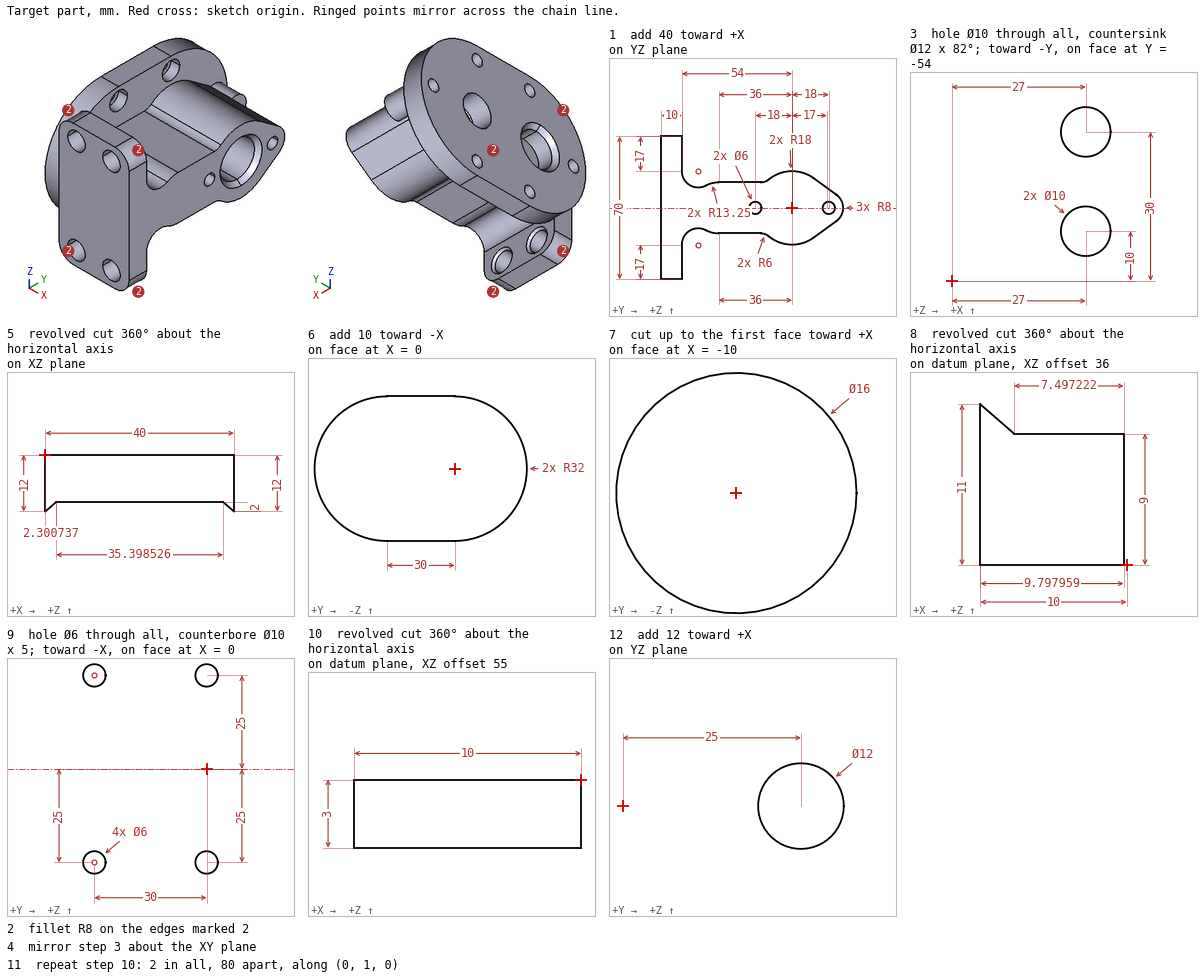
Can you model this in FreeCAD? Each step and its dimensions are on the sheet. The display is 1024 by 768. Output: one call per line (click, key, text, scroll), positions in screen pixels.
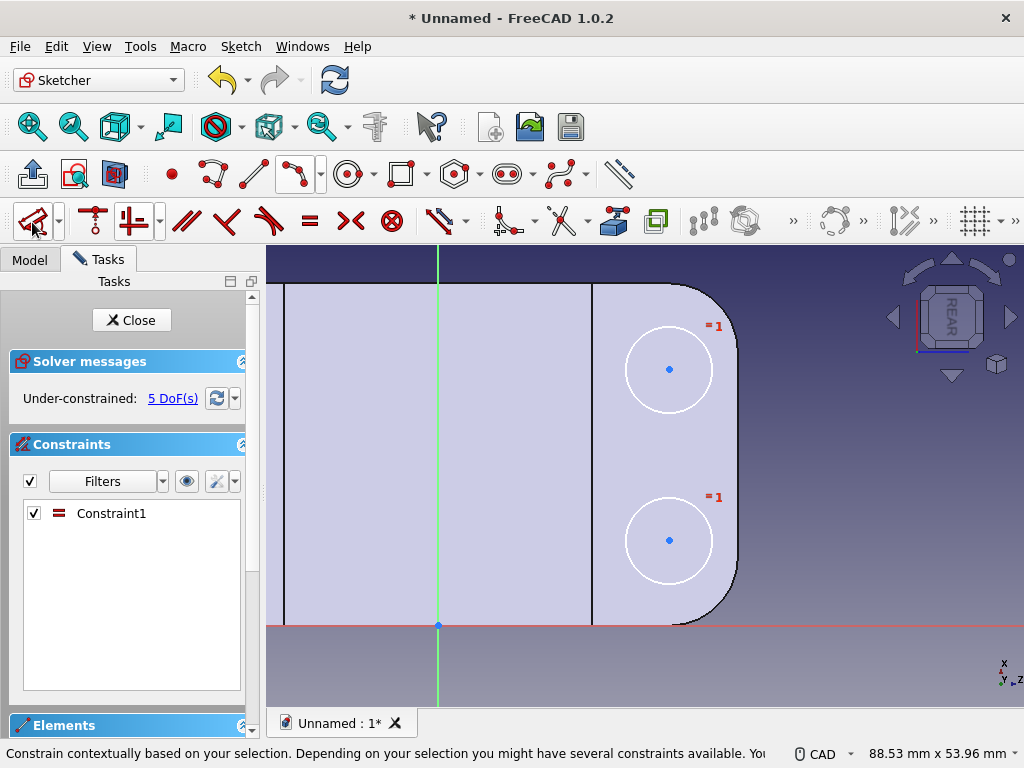
click(699, 510)
click(721, 487)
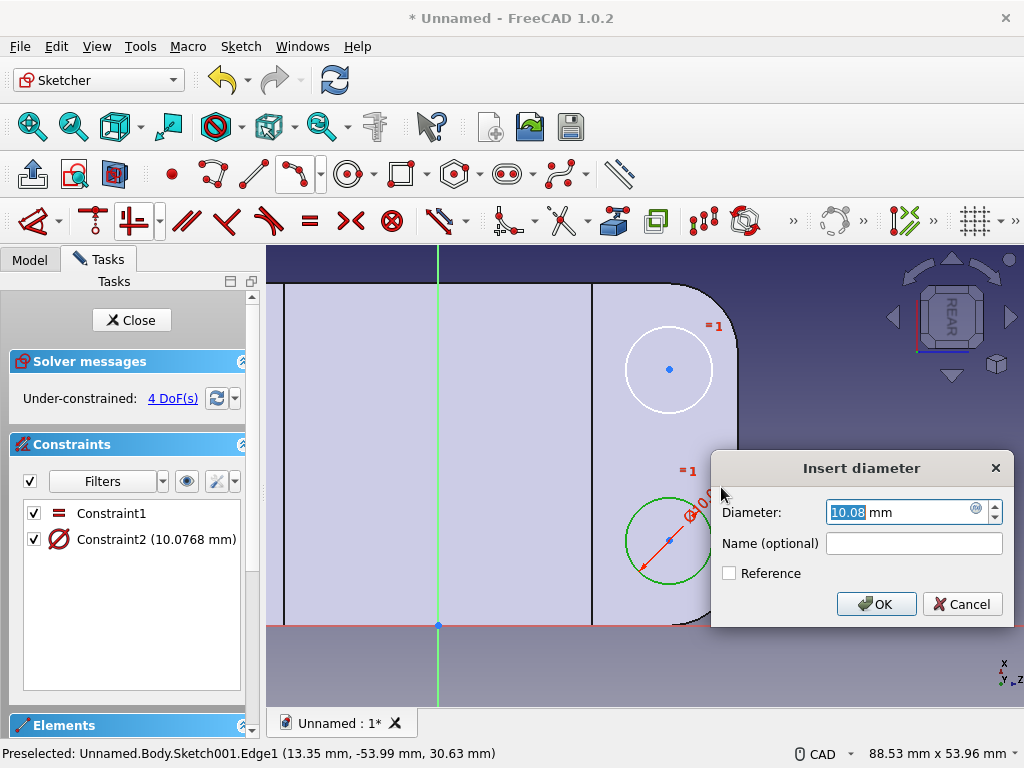
text(10)
key(Return)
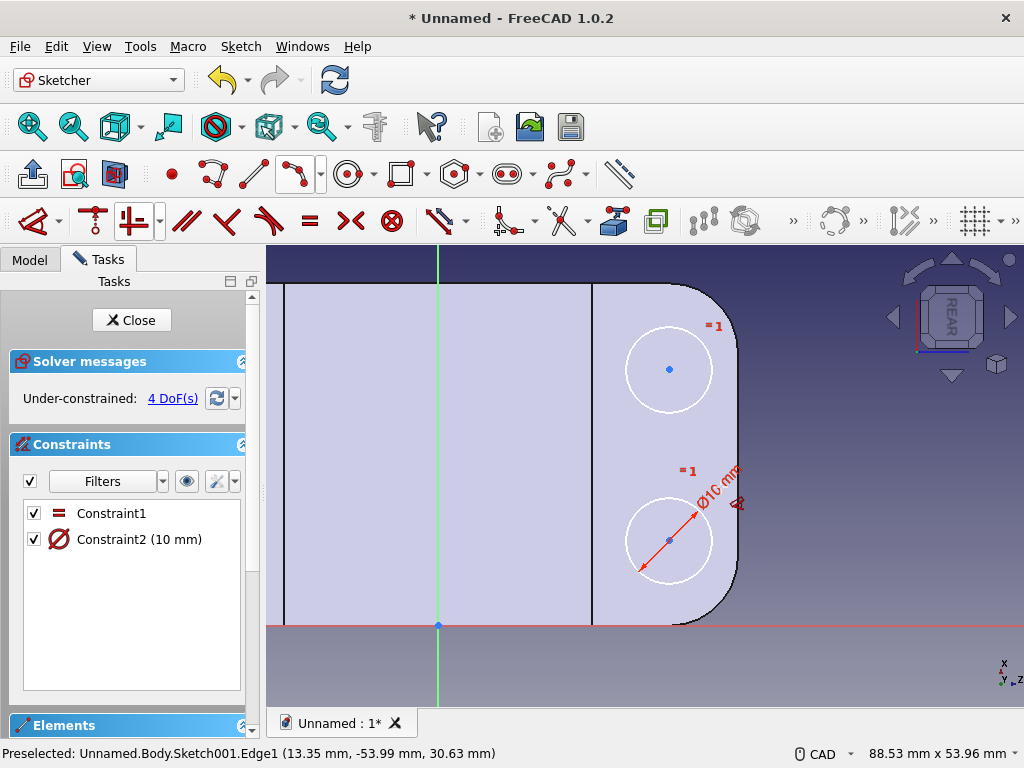
click(669, 541)
click(554, 660)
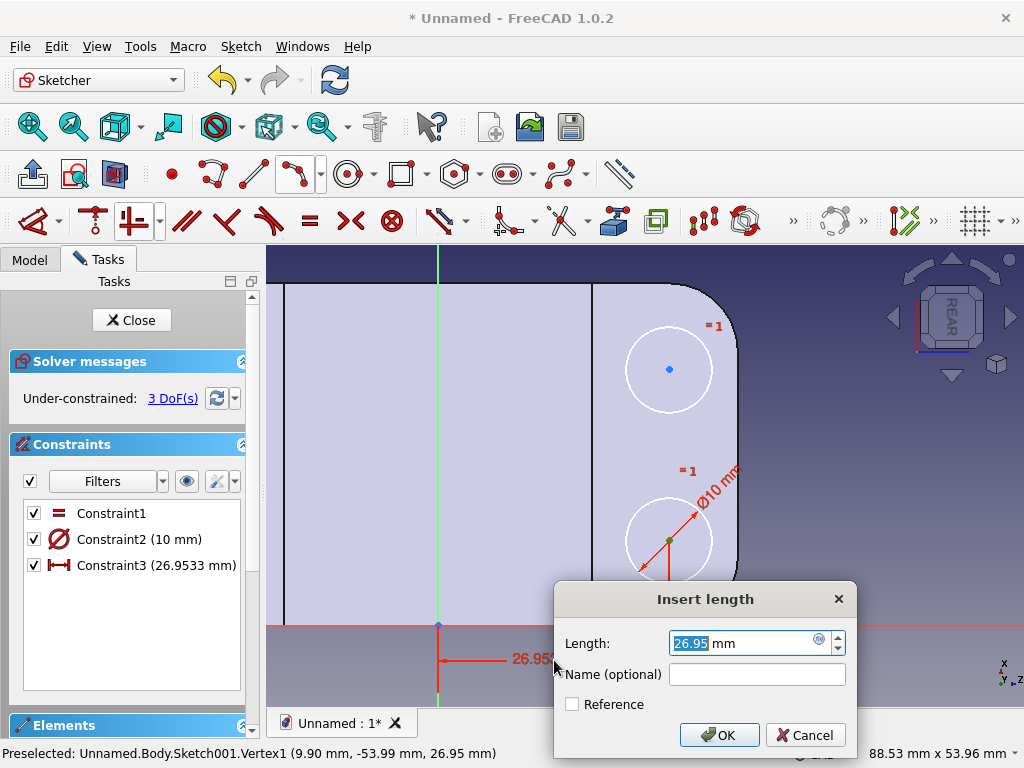
text(27)
key(Return)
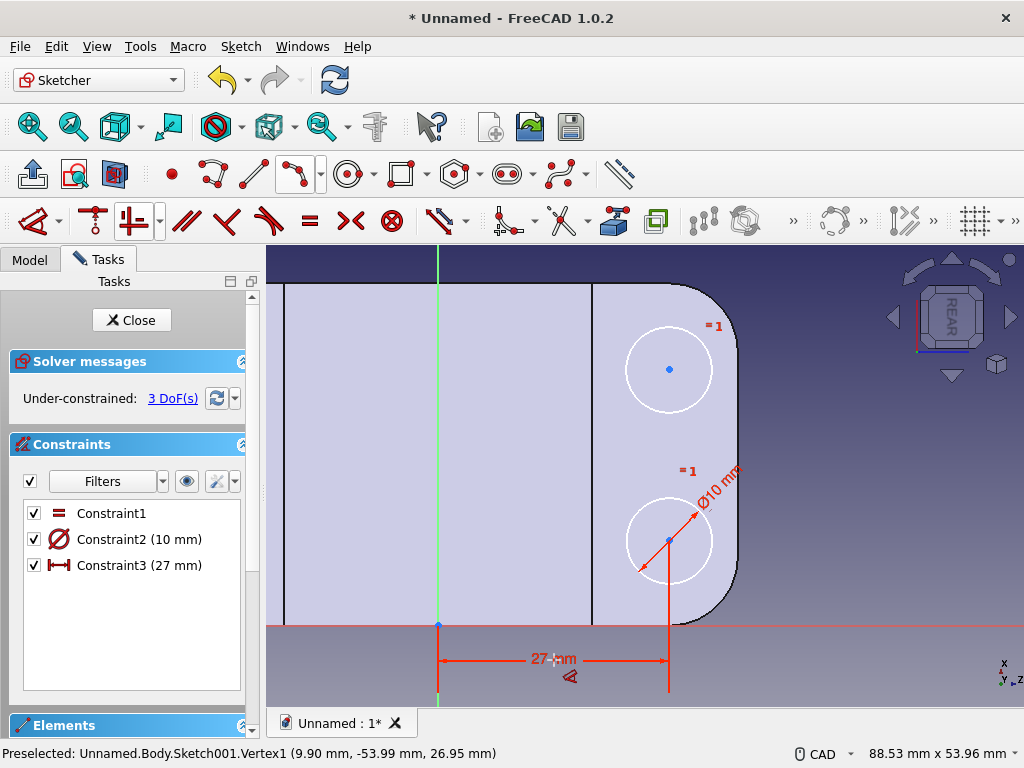
click(669, 541)
click(404, 583)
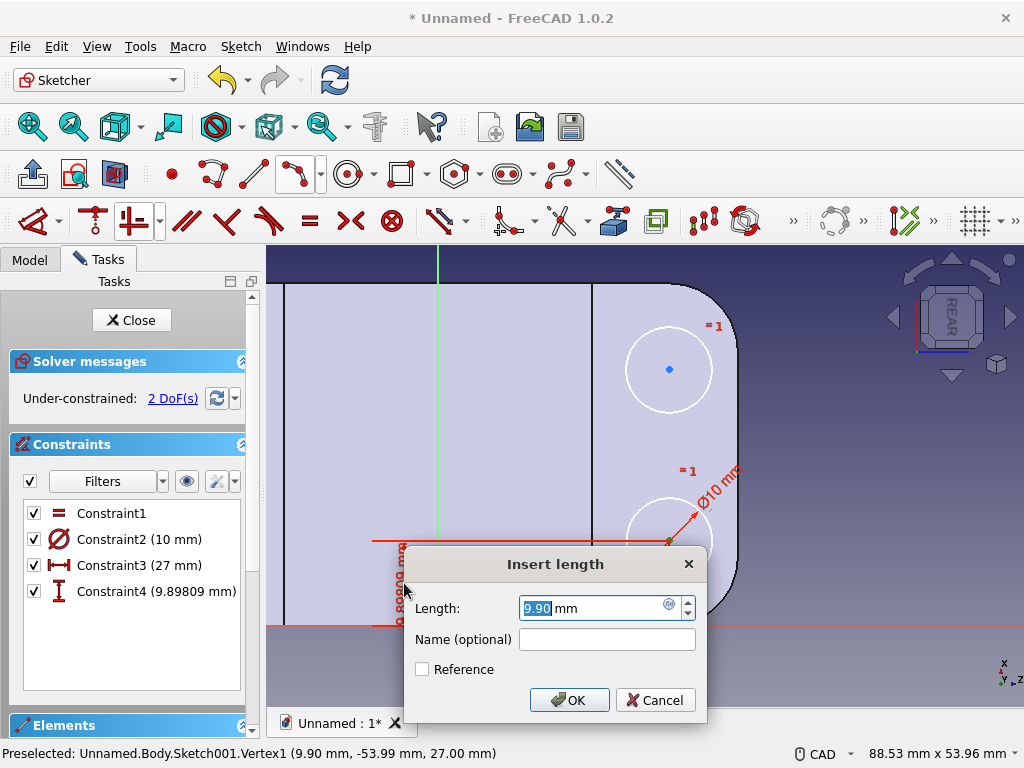
text(10)
key(Return)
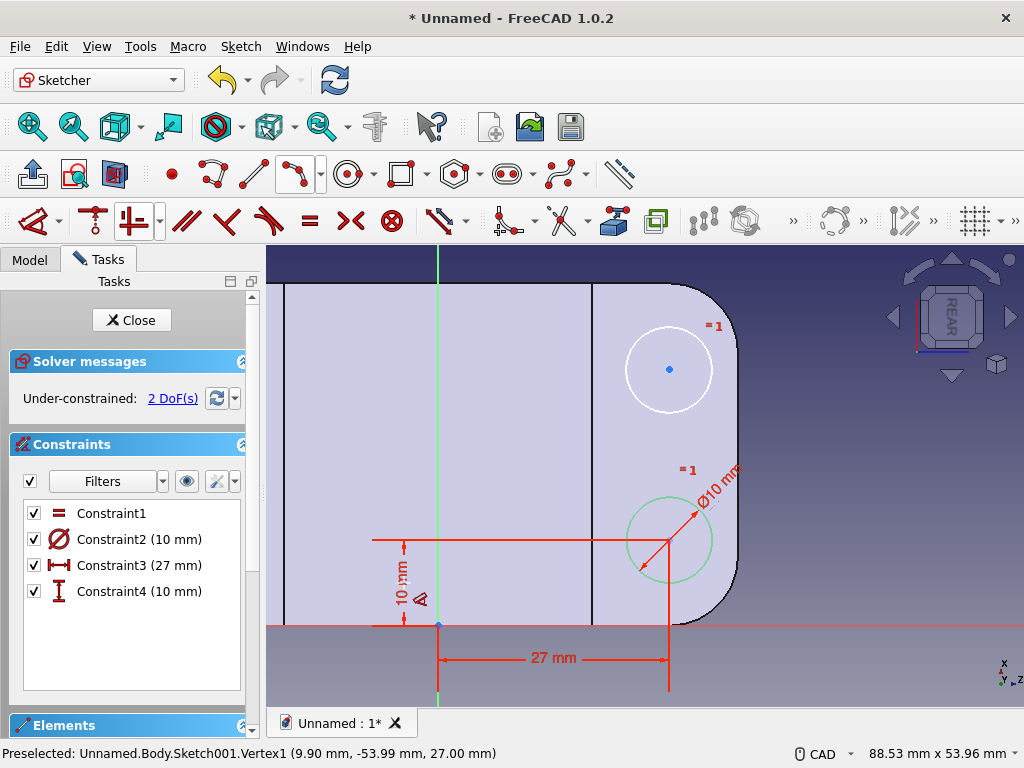
click(669, 370)
click(473, 660)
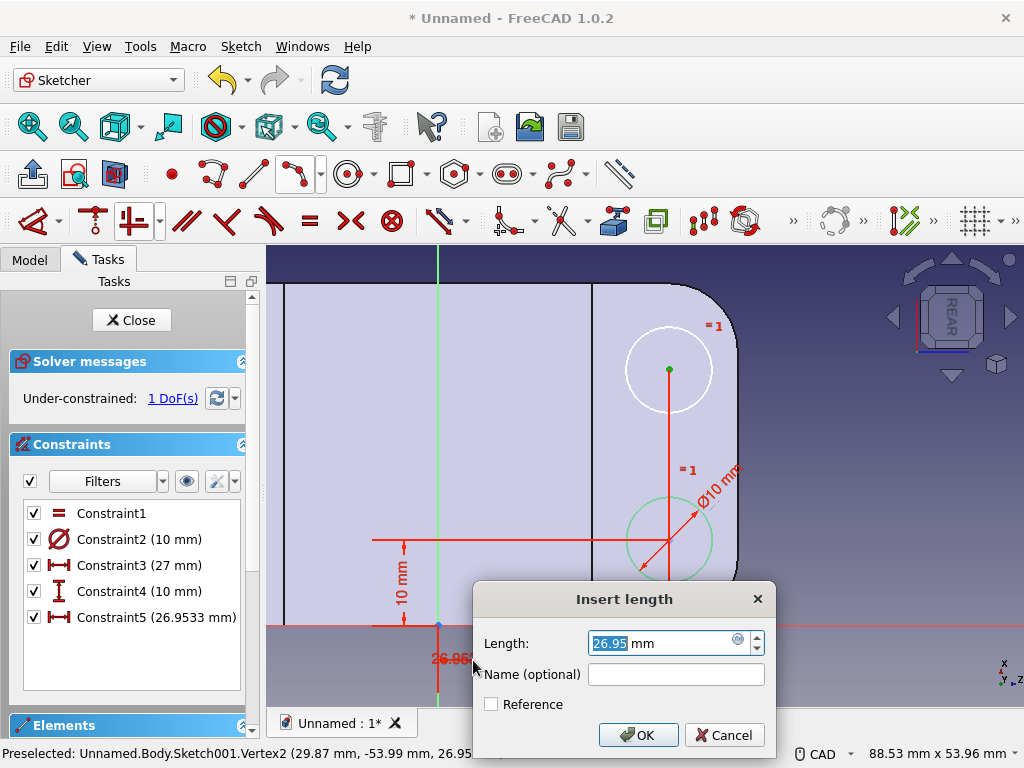
text(27)
key(Return)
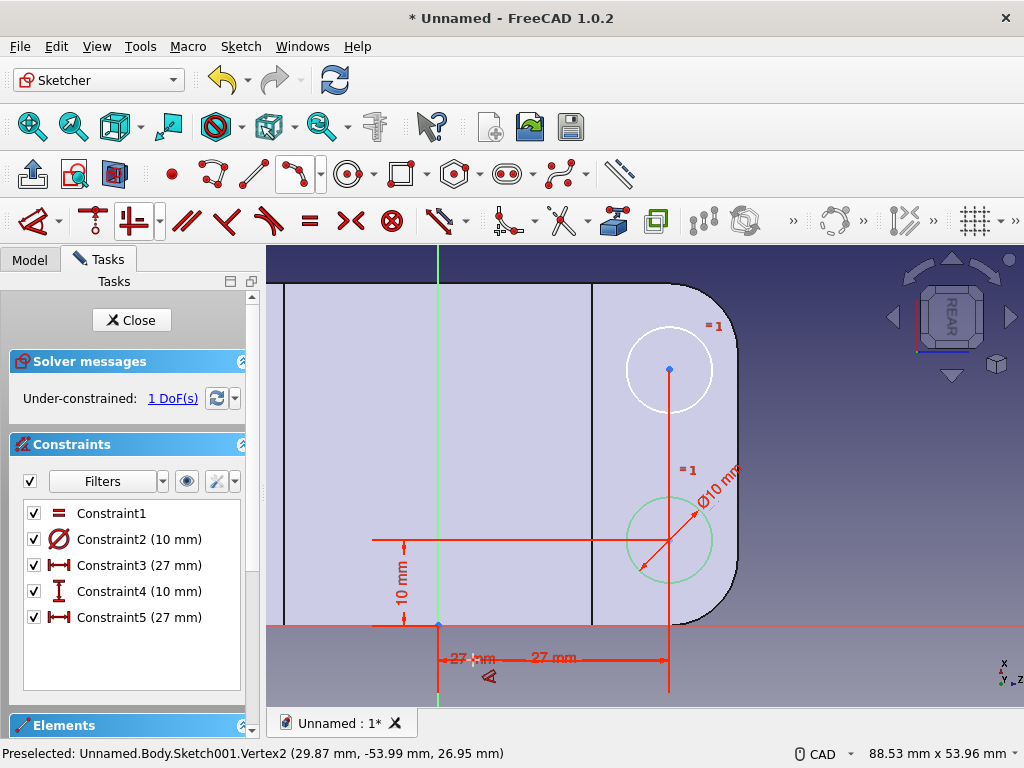
click(669, 370)
click(404, 498)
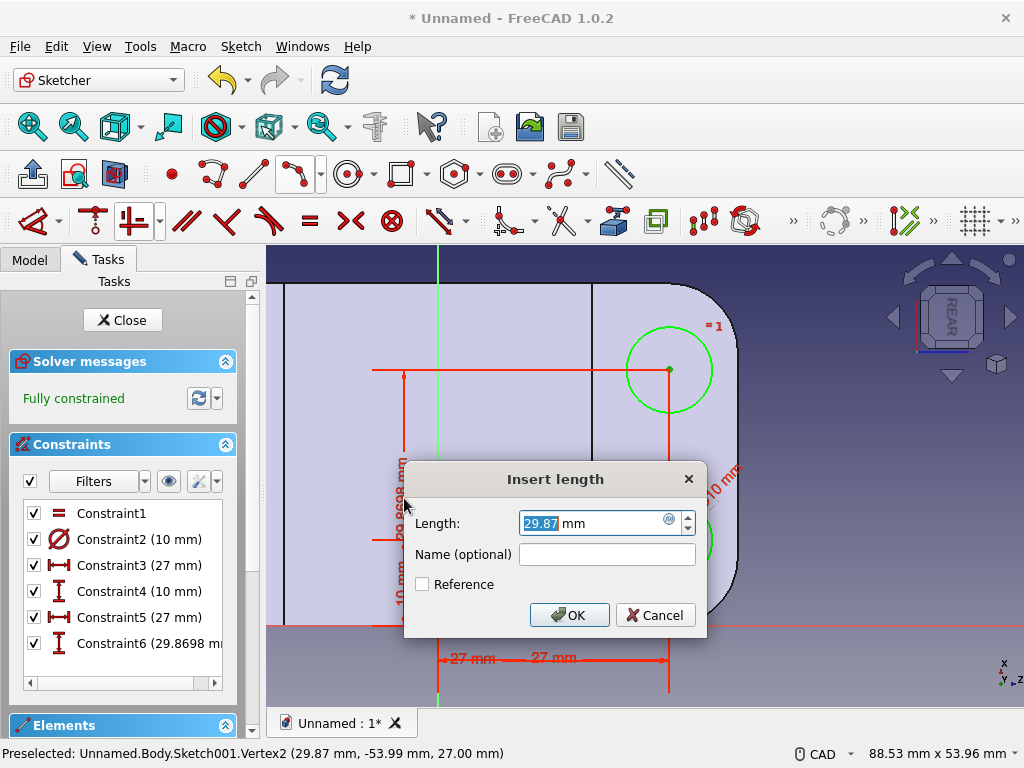
text(30)
key(Return)
key(Escape)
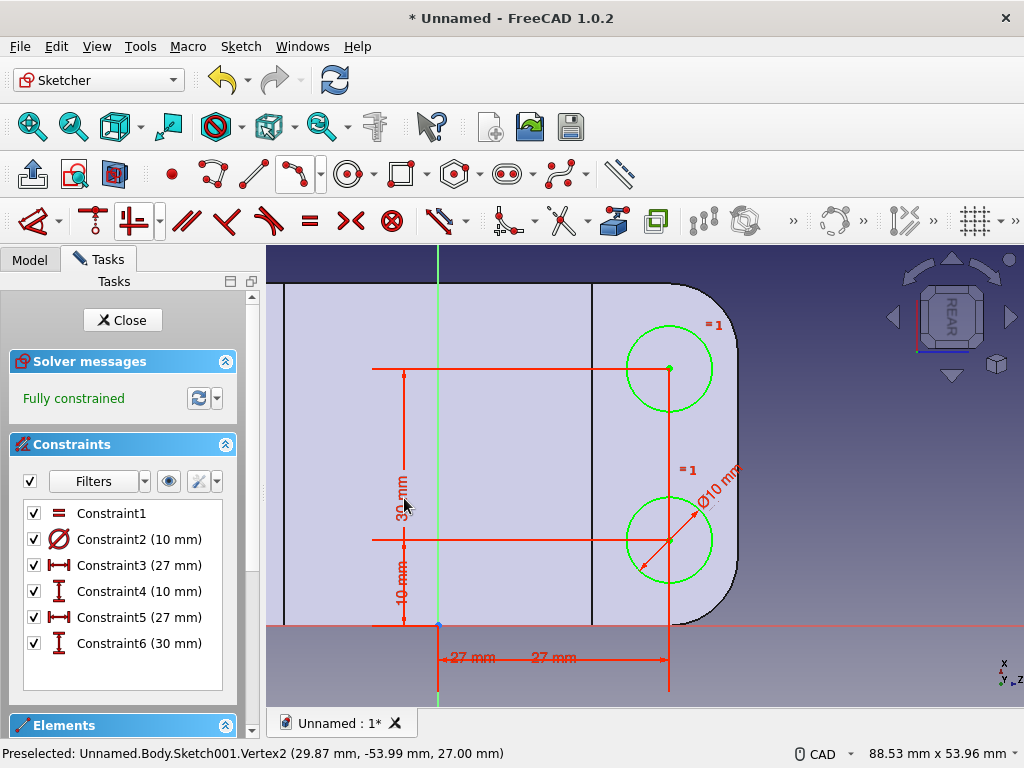
click(123, 320)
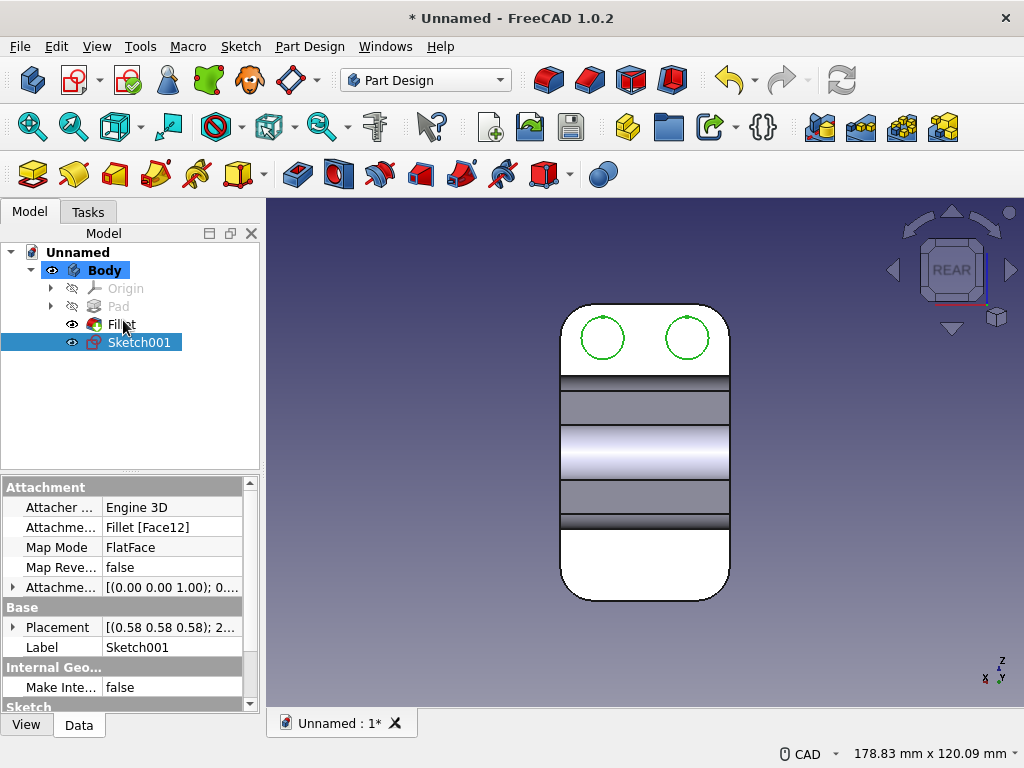
click(339, 174)